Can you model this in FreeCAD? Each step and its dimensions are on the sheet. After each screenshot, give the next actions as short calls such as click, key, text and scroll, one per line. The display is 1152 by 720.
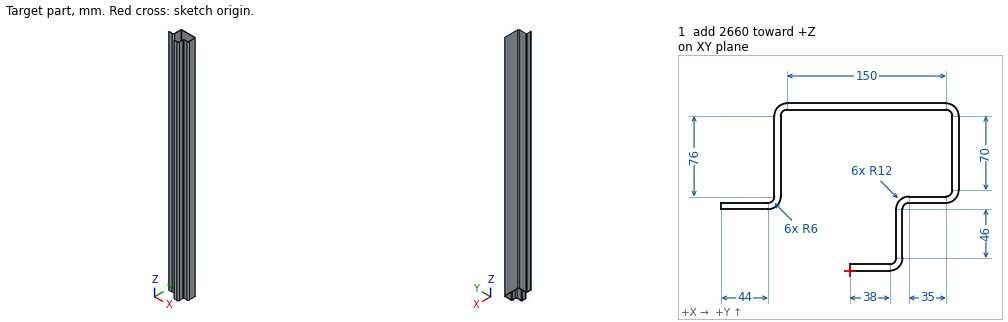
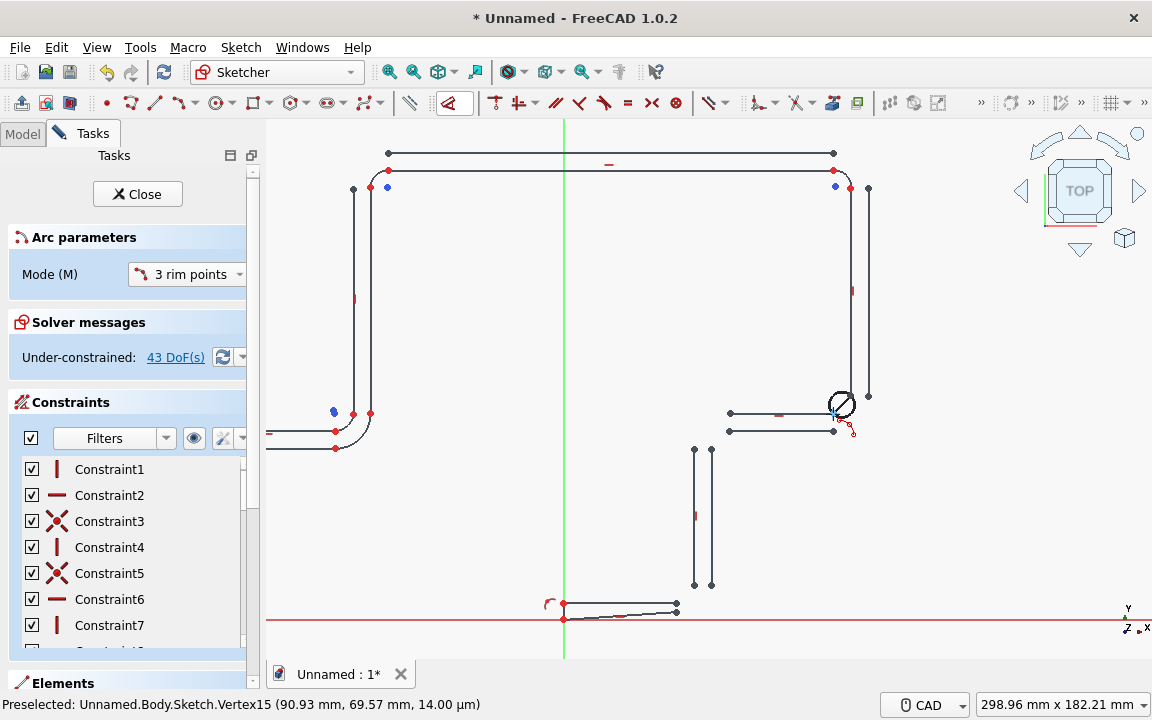
scroll(846, 407, up, 6)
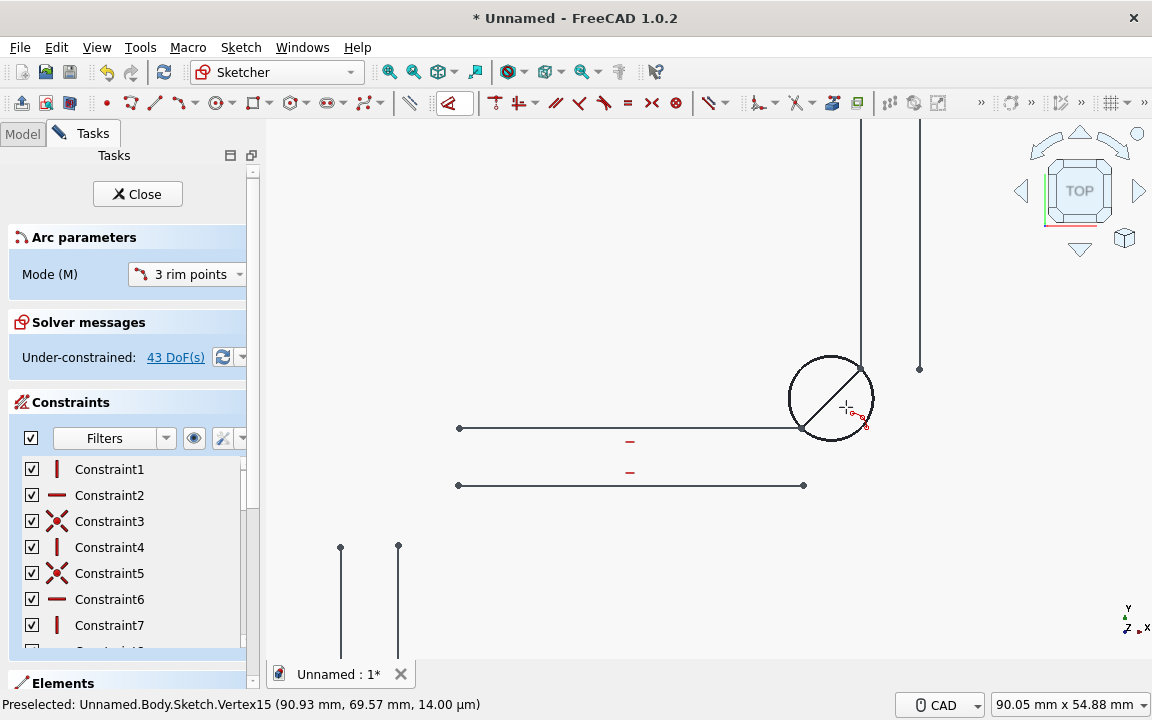
click(844, 407)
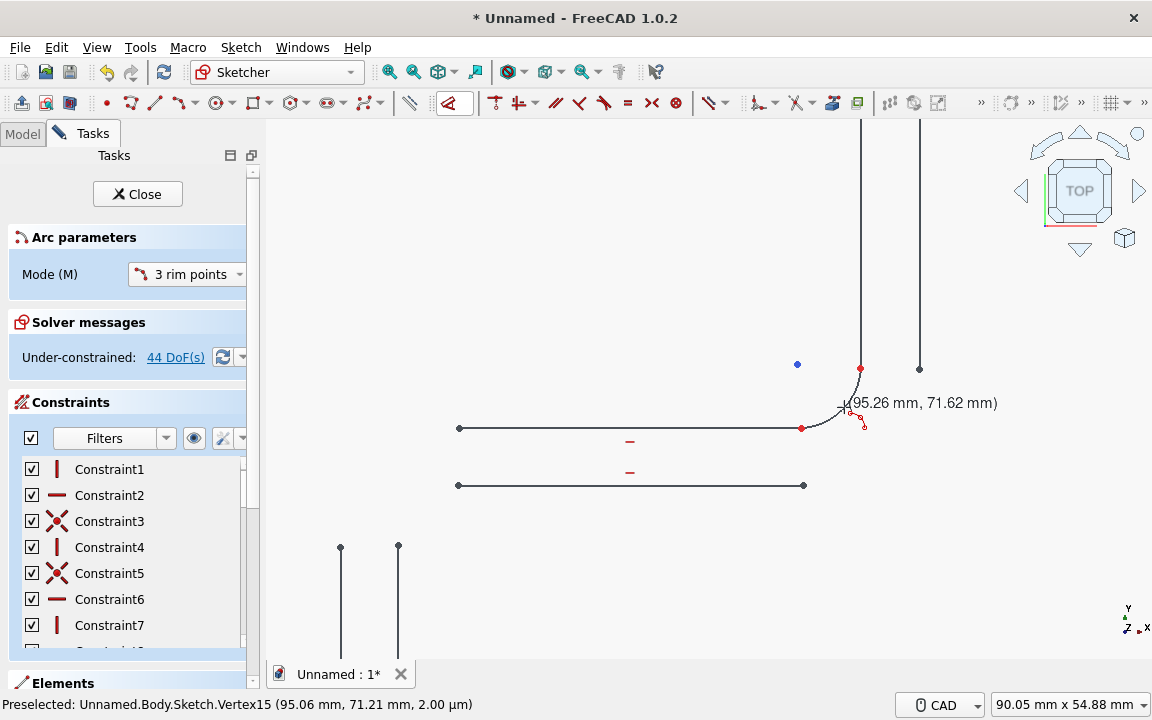
scroll(849, 403, down, 8)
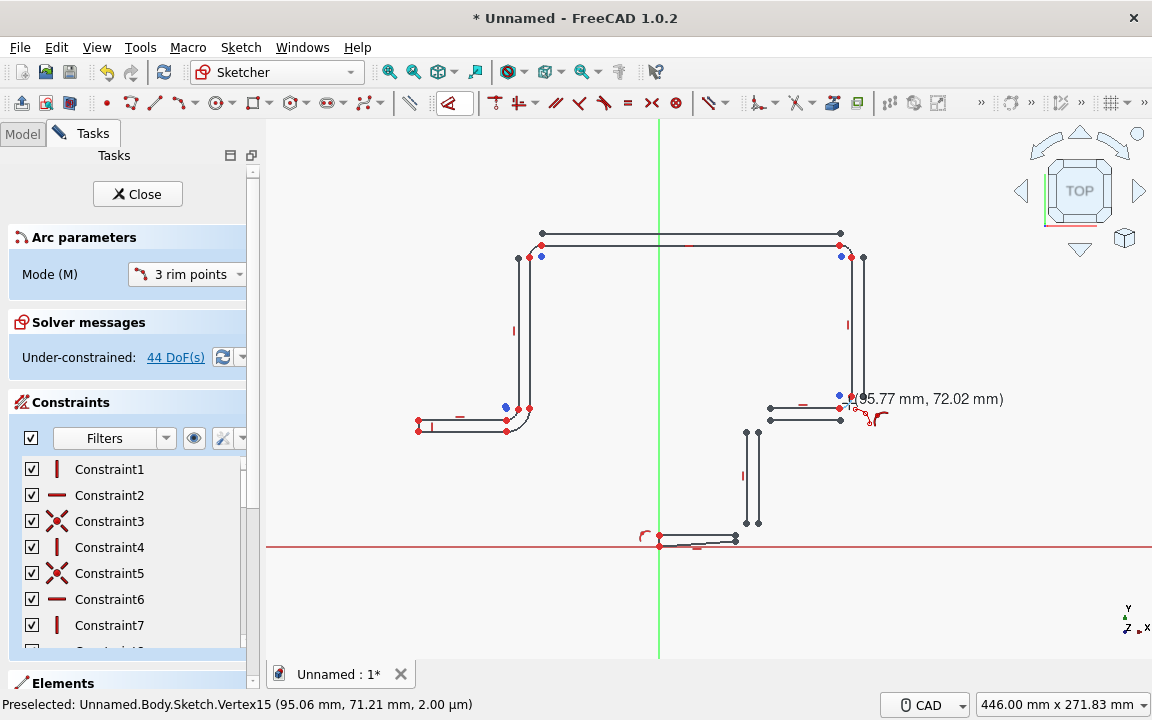
scroll(771, 408, up, 2)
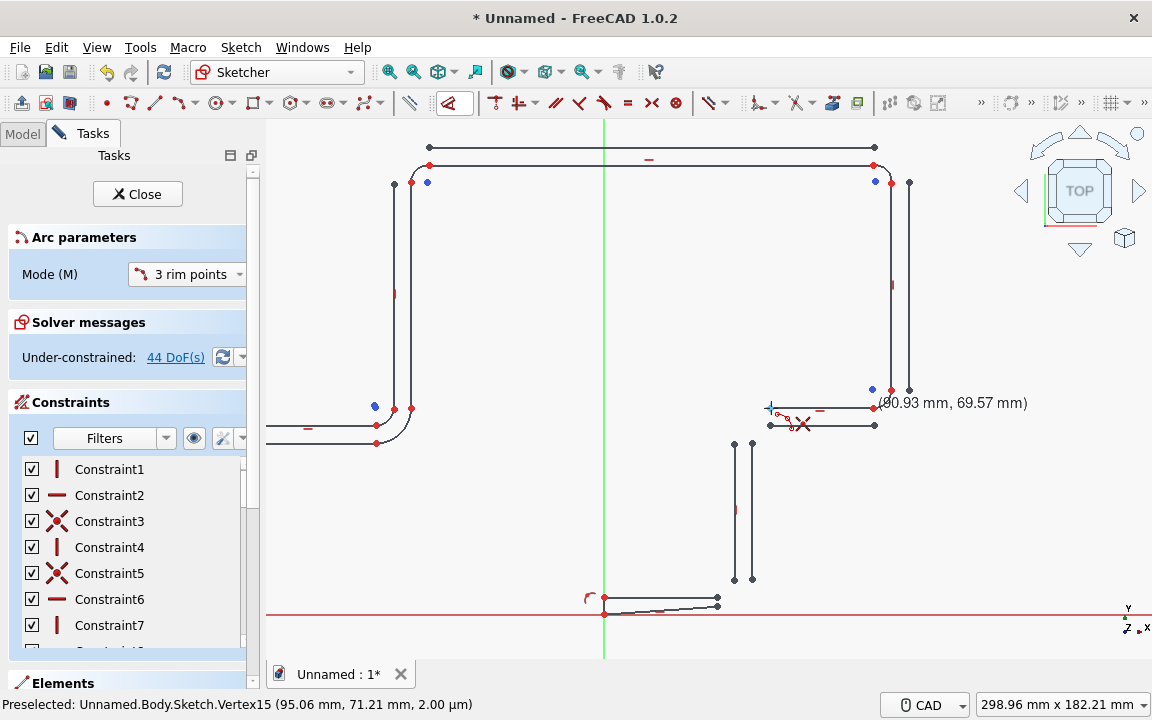
click(771, 408)
click(735, 444)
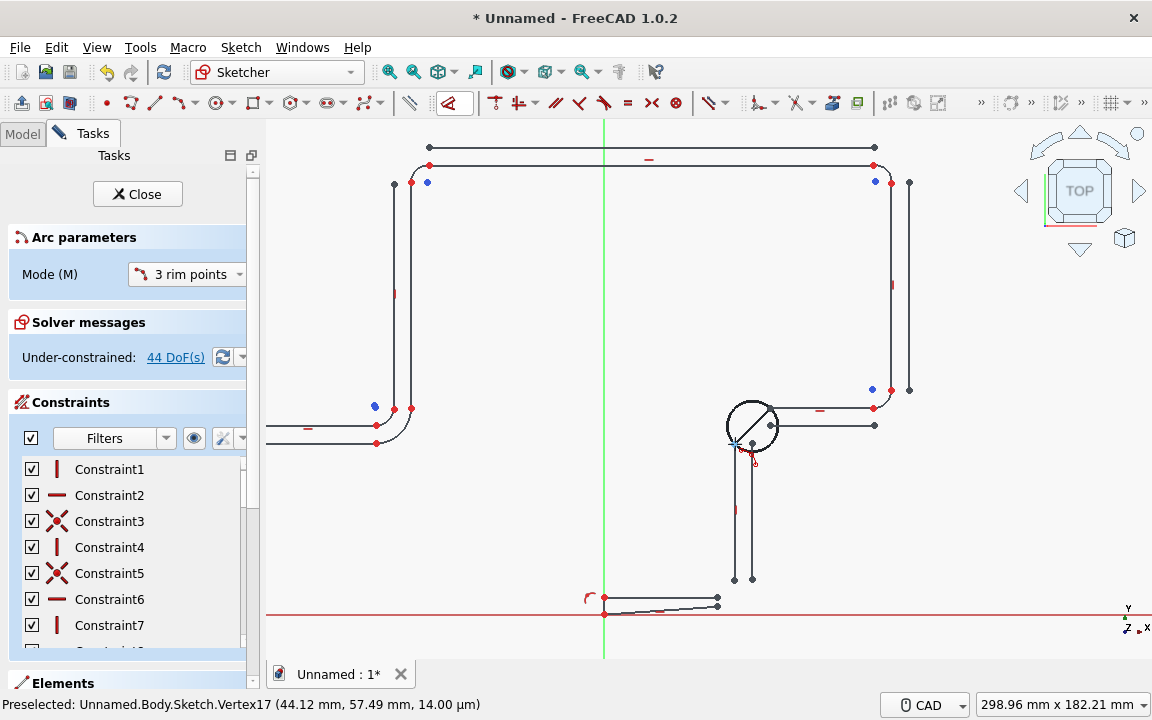
scroll(745, 418, up, 3)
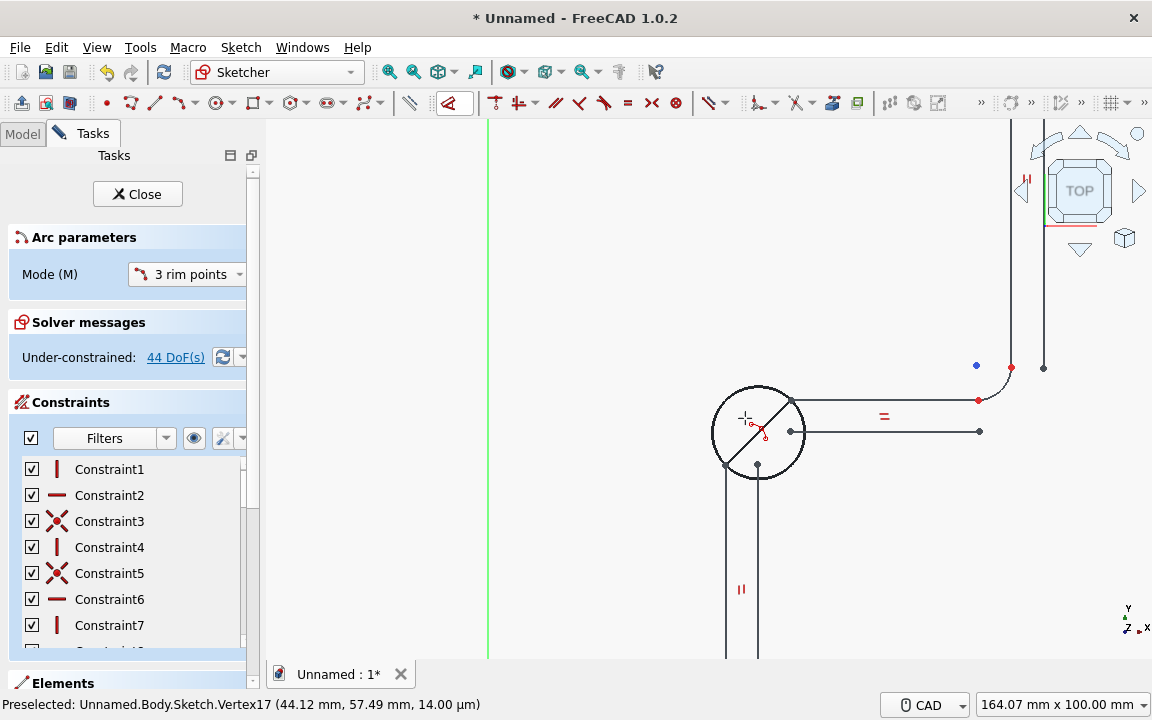
click(744, 417)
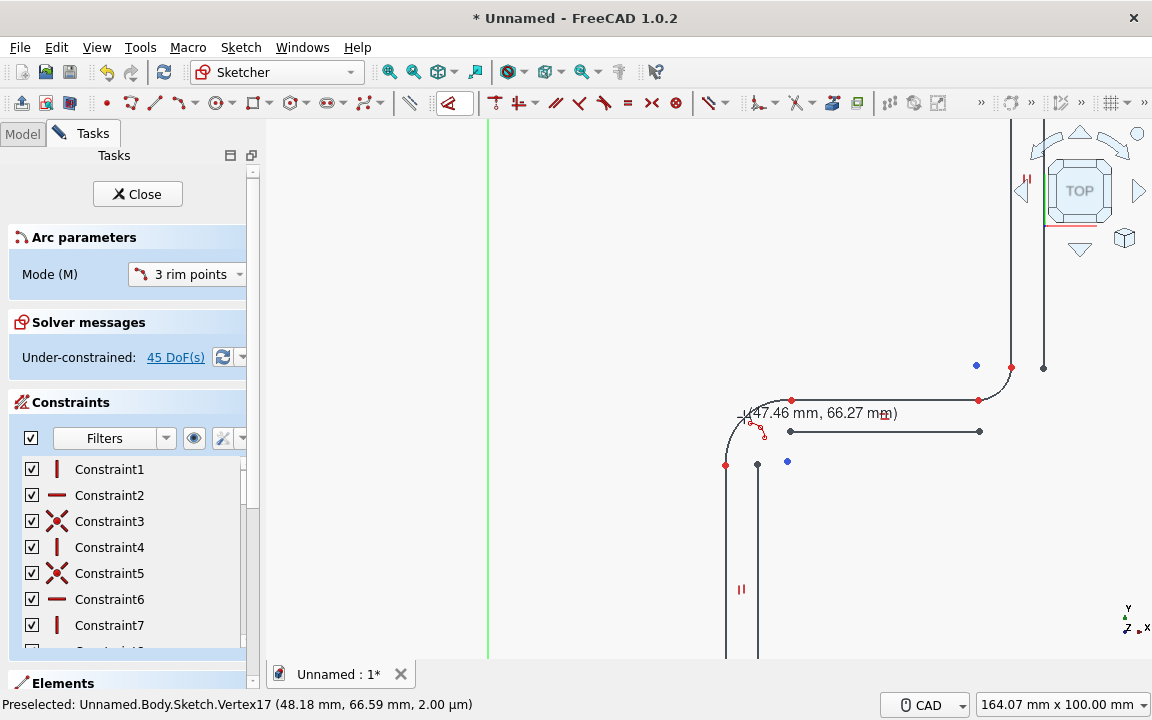
scroll(758, 412, down, 5)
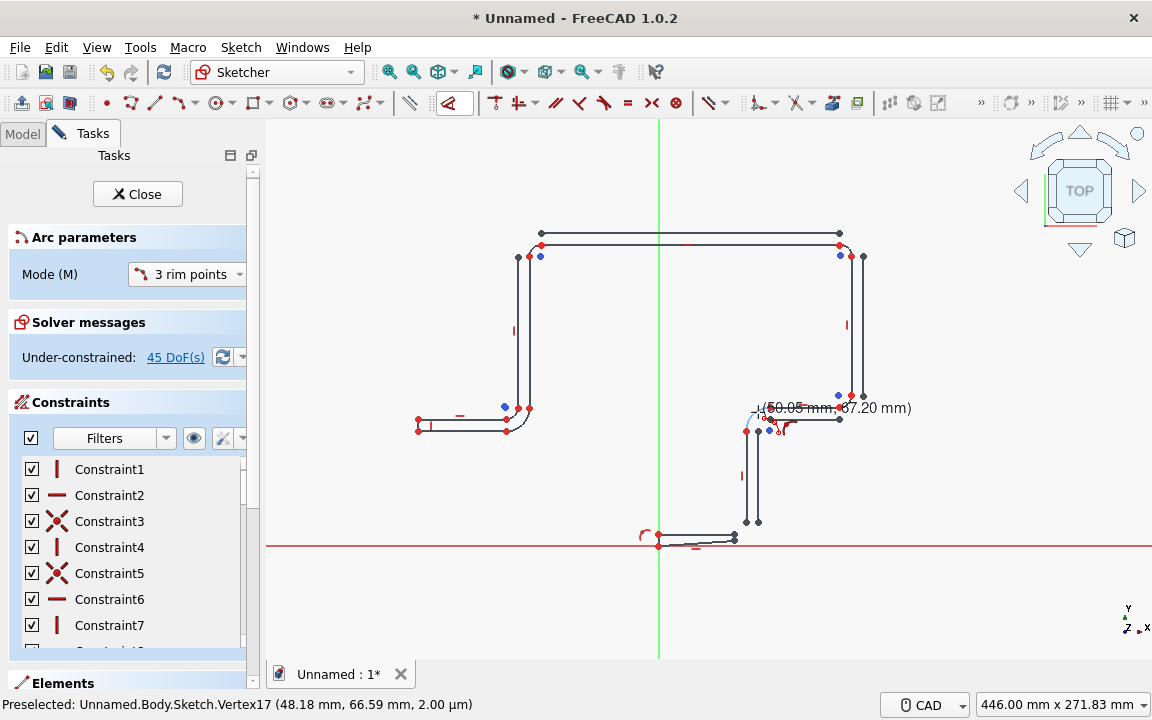
scroll(746, 522, up, 2)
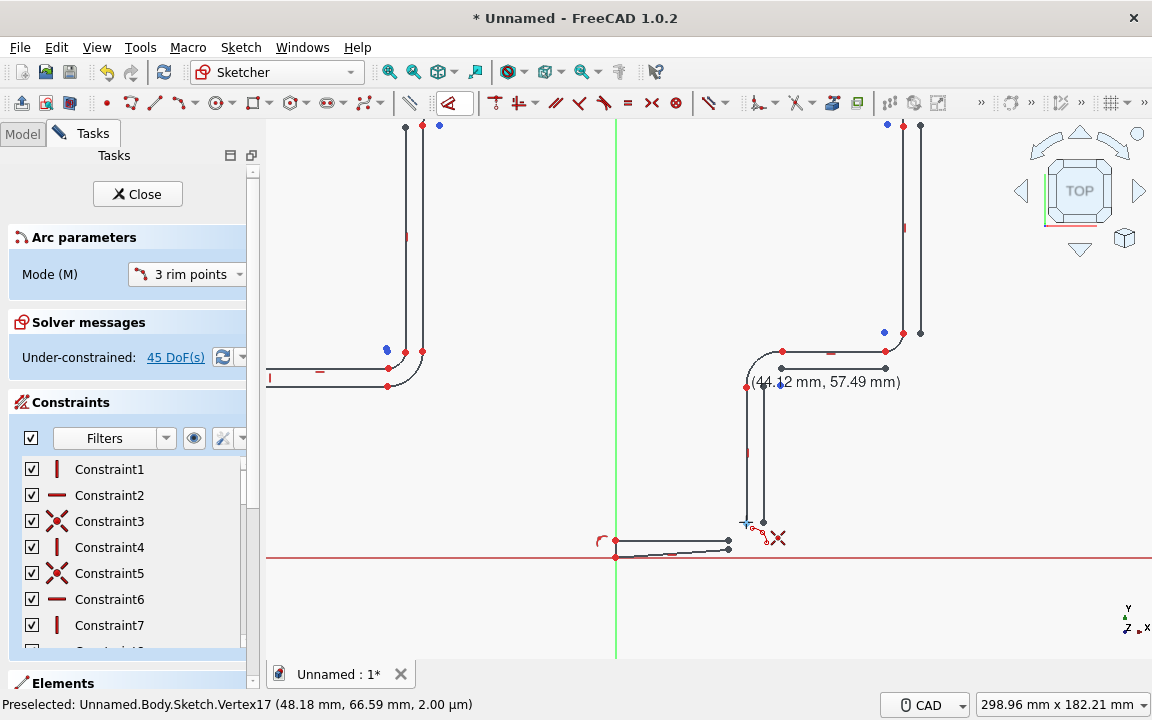
click(747, 523)
click(729, 541)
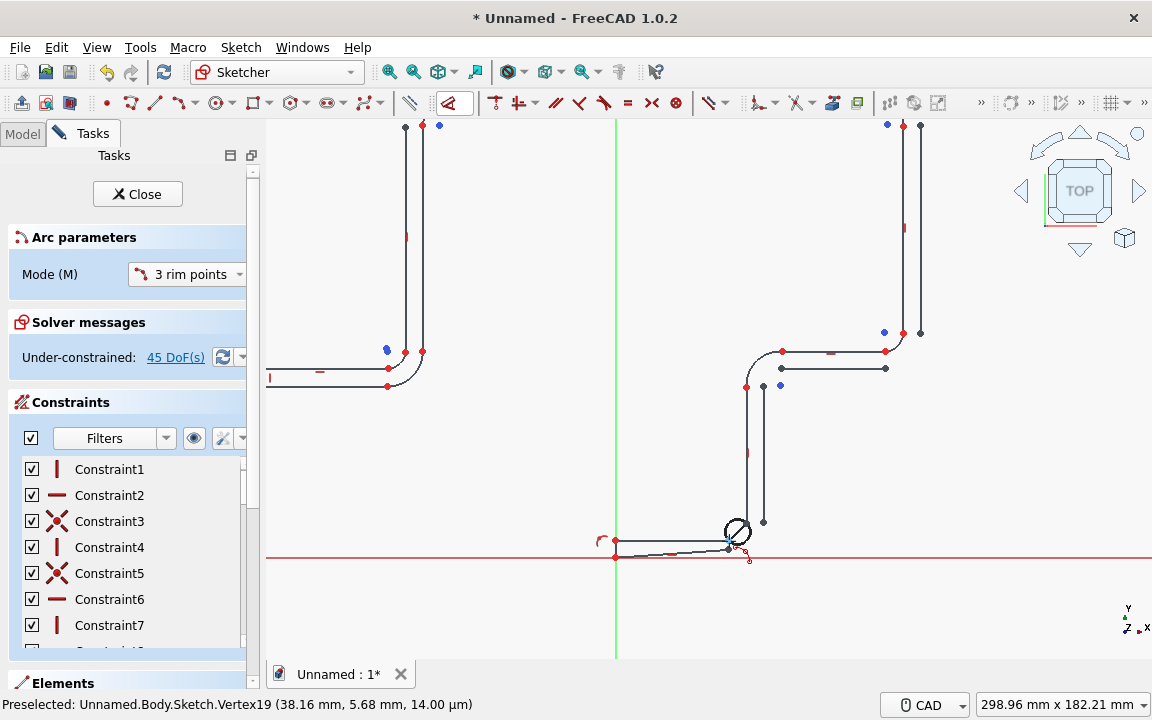
scroll(741, 535, up, 6)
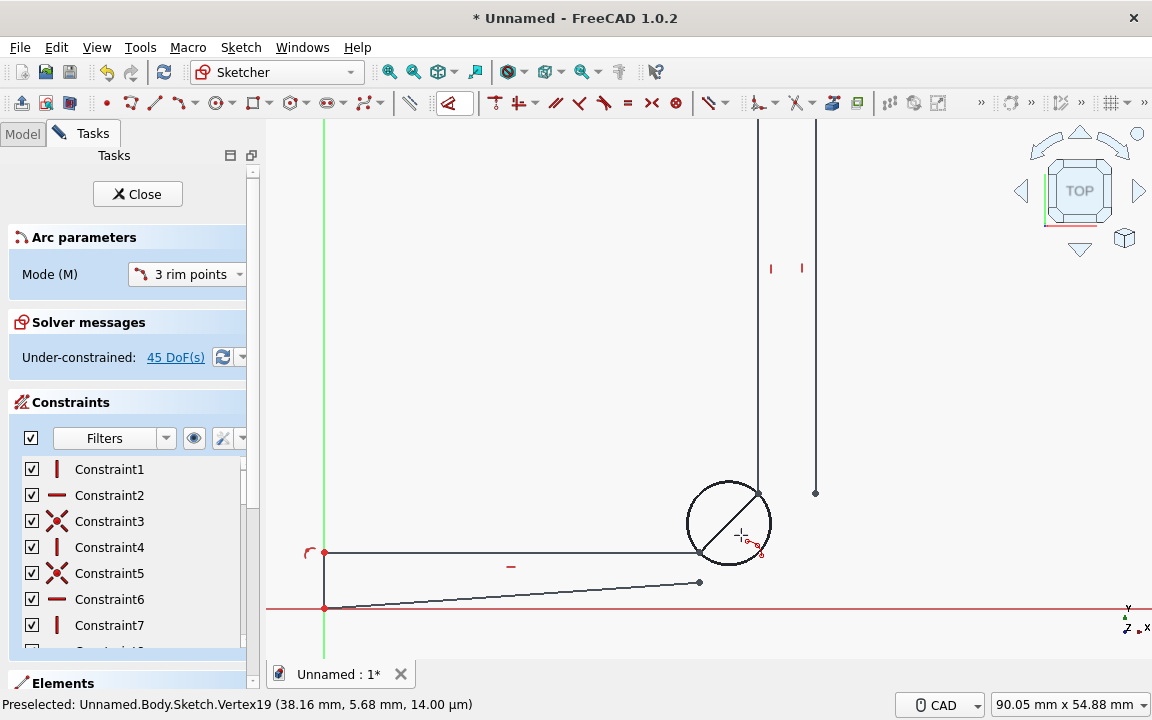
click(740, 532)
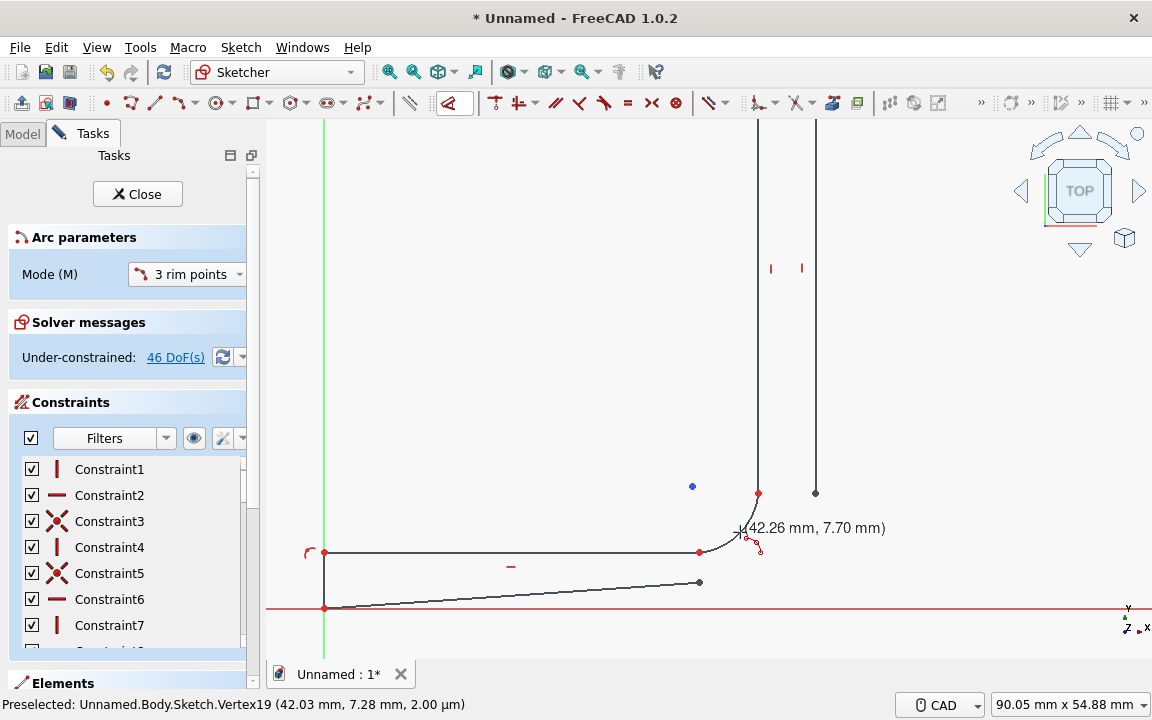
scroll(743, 530, down, 8)